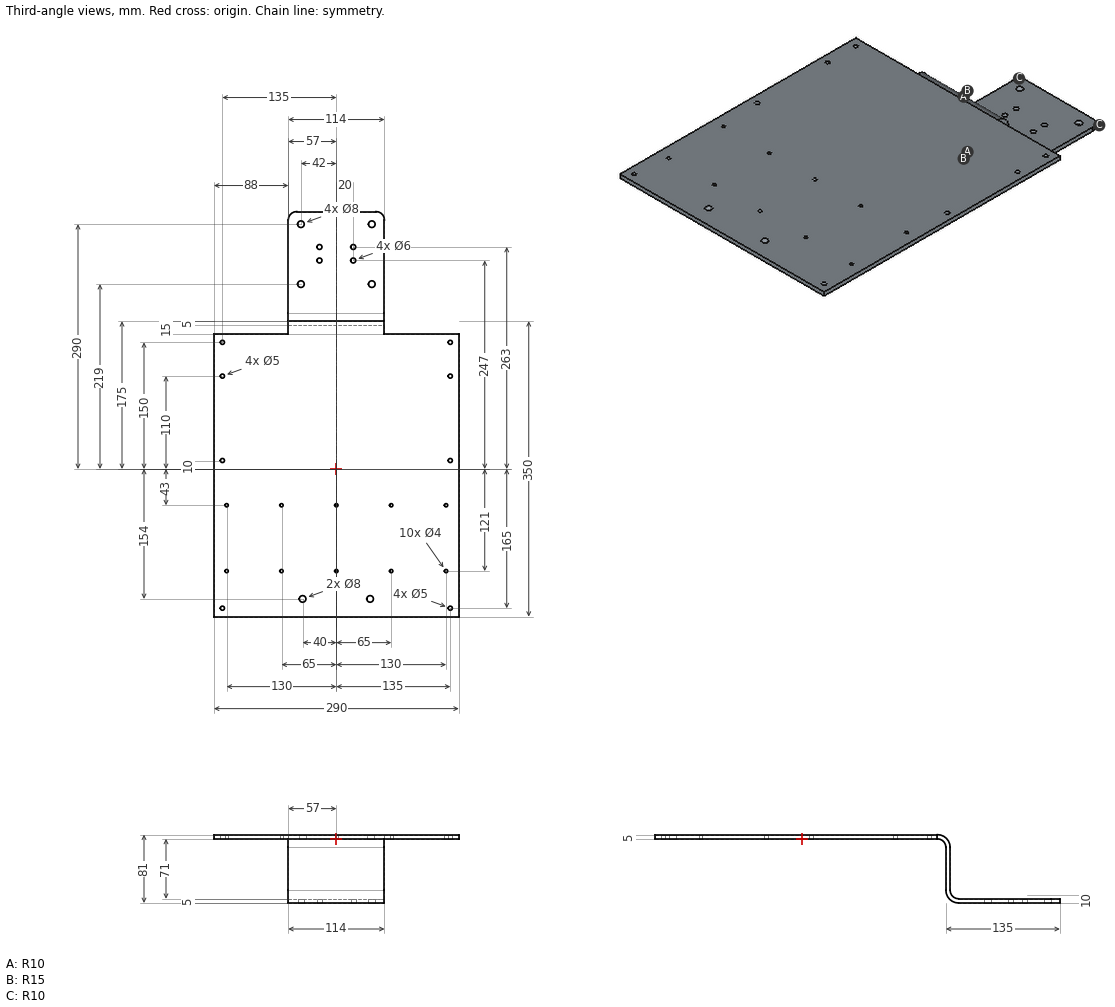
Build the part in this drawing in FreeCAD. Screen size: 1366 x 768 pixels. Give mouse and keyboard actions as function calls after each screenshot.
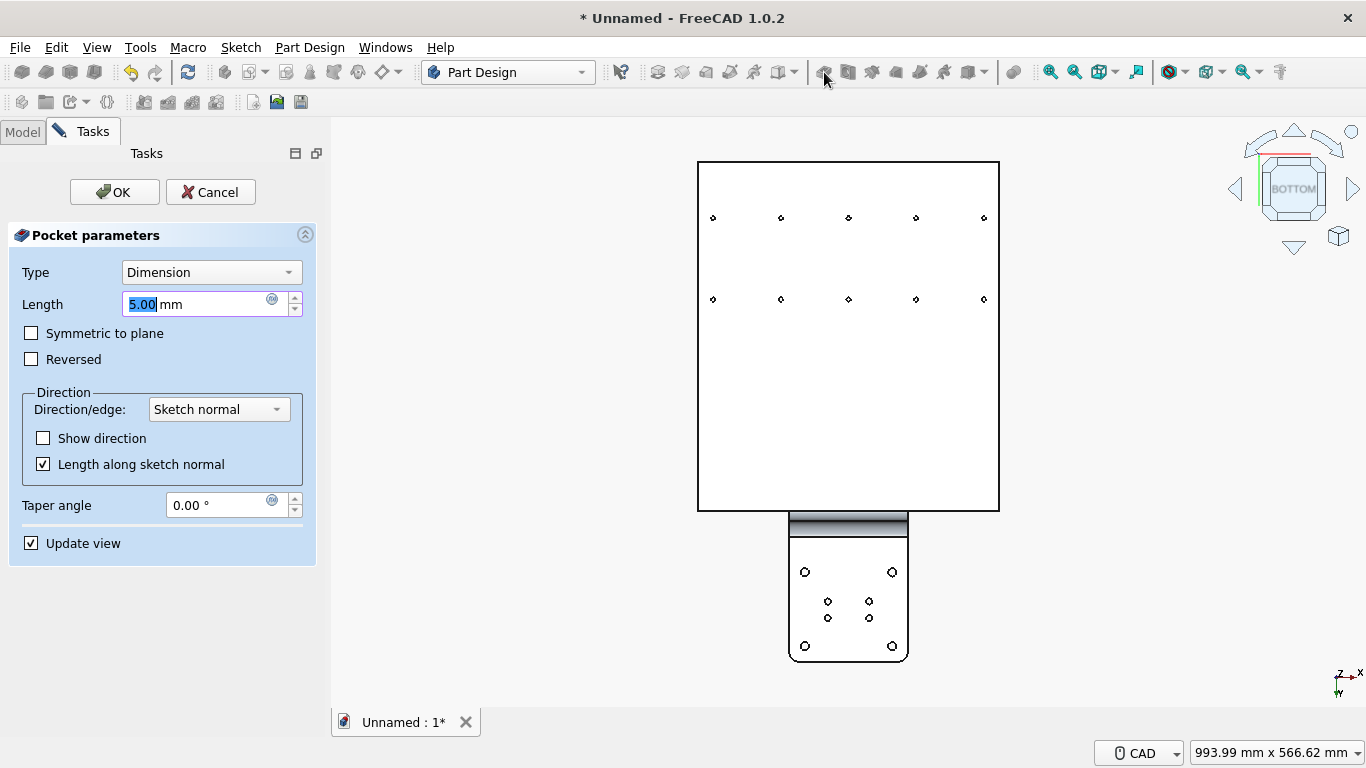
text(10)
key(Tab)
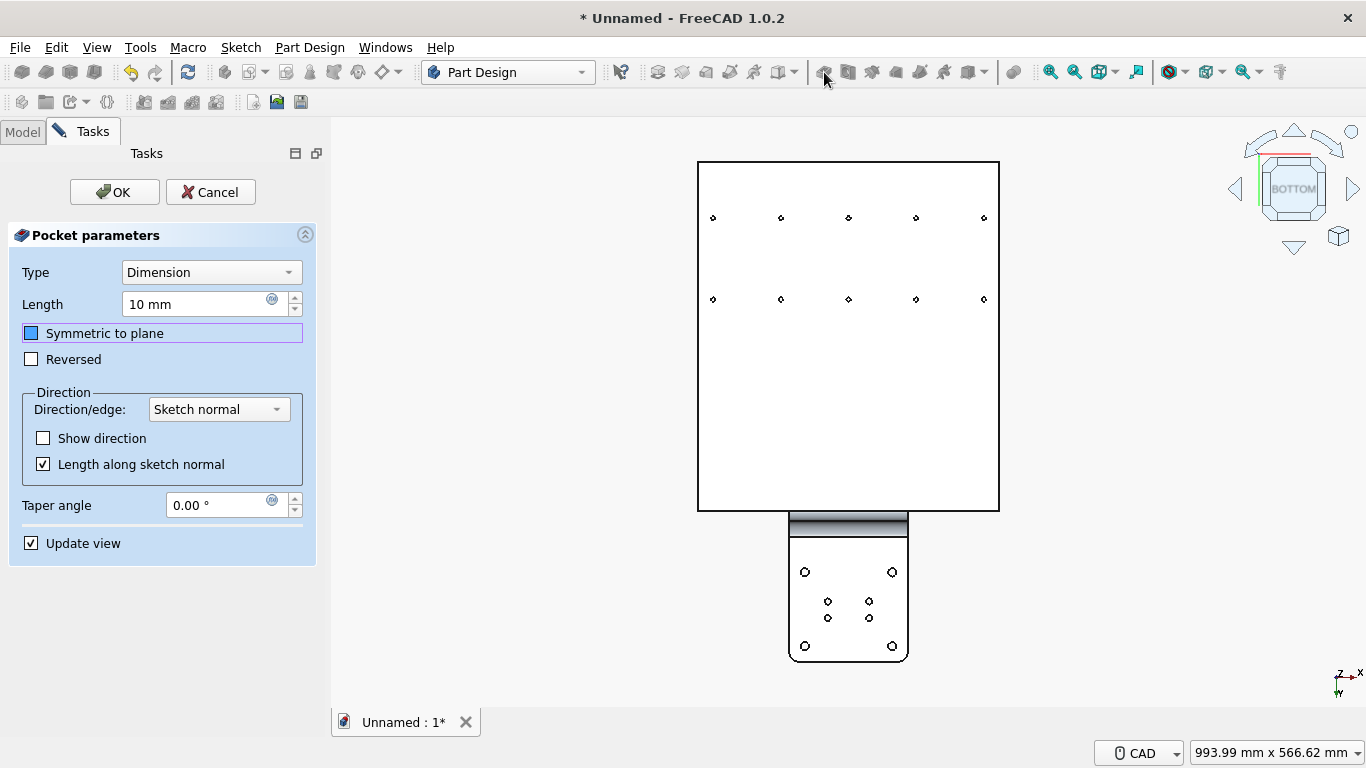
click(115, 192)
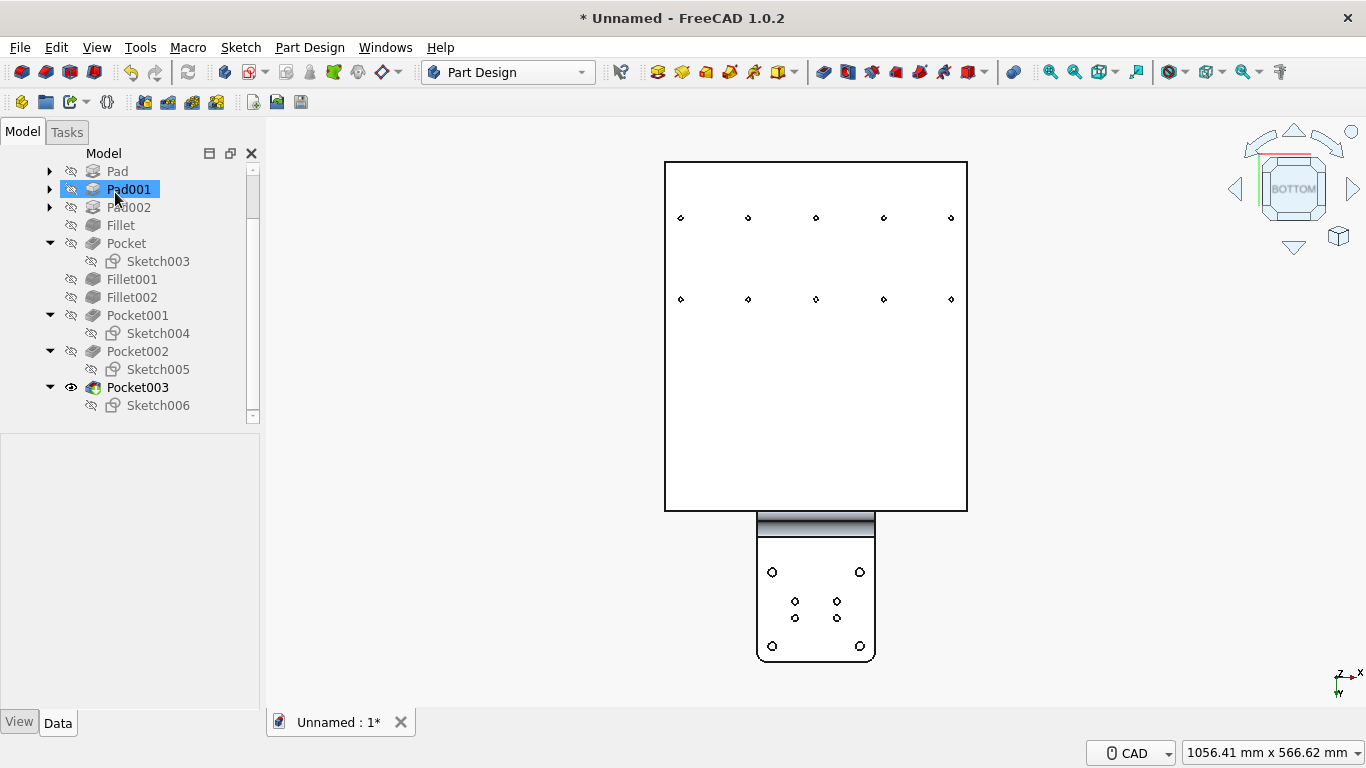
click(250, 72)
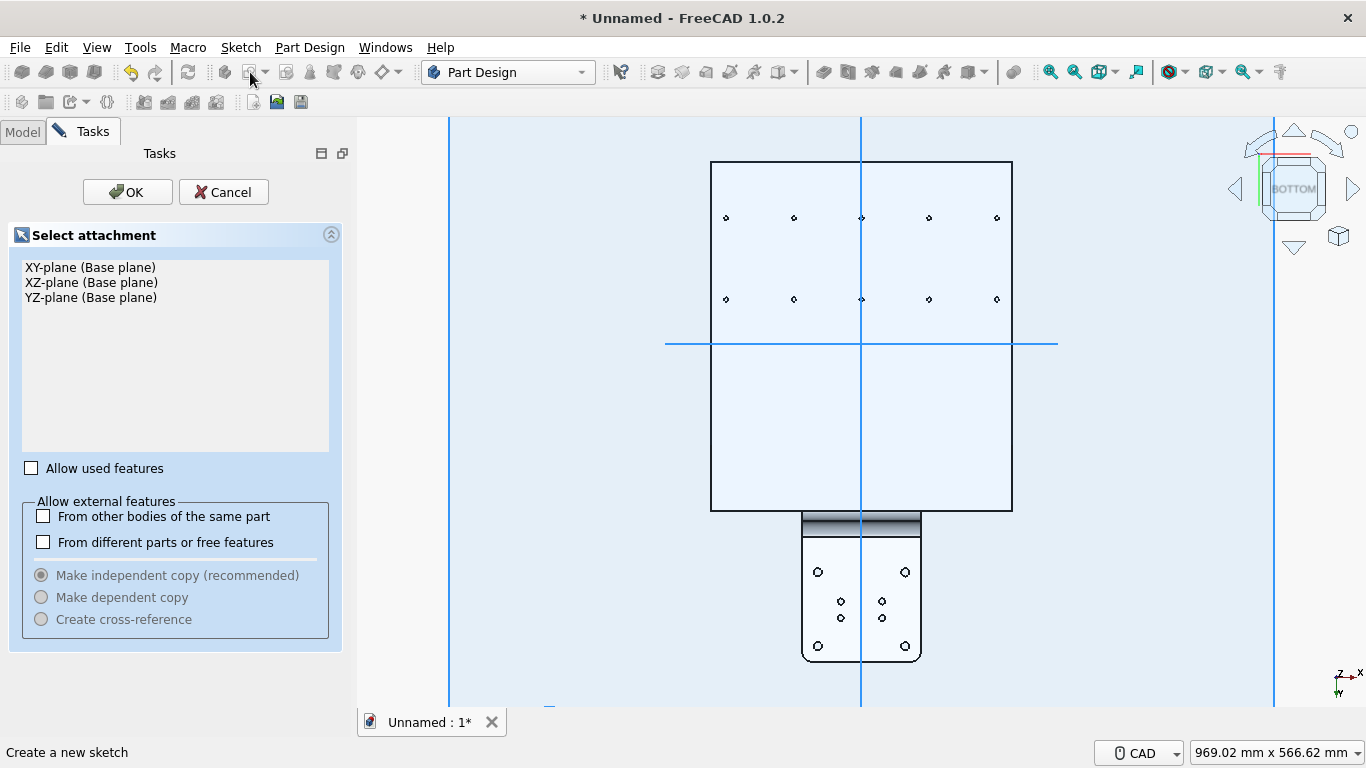
click(82, 268)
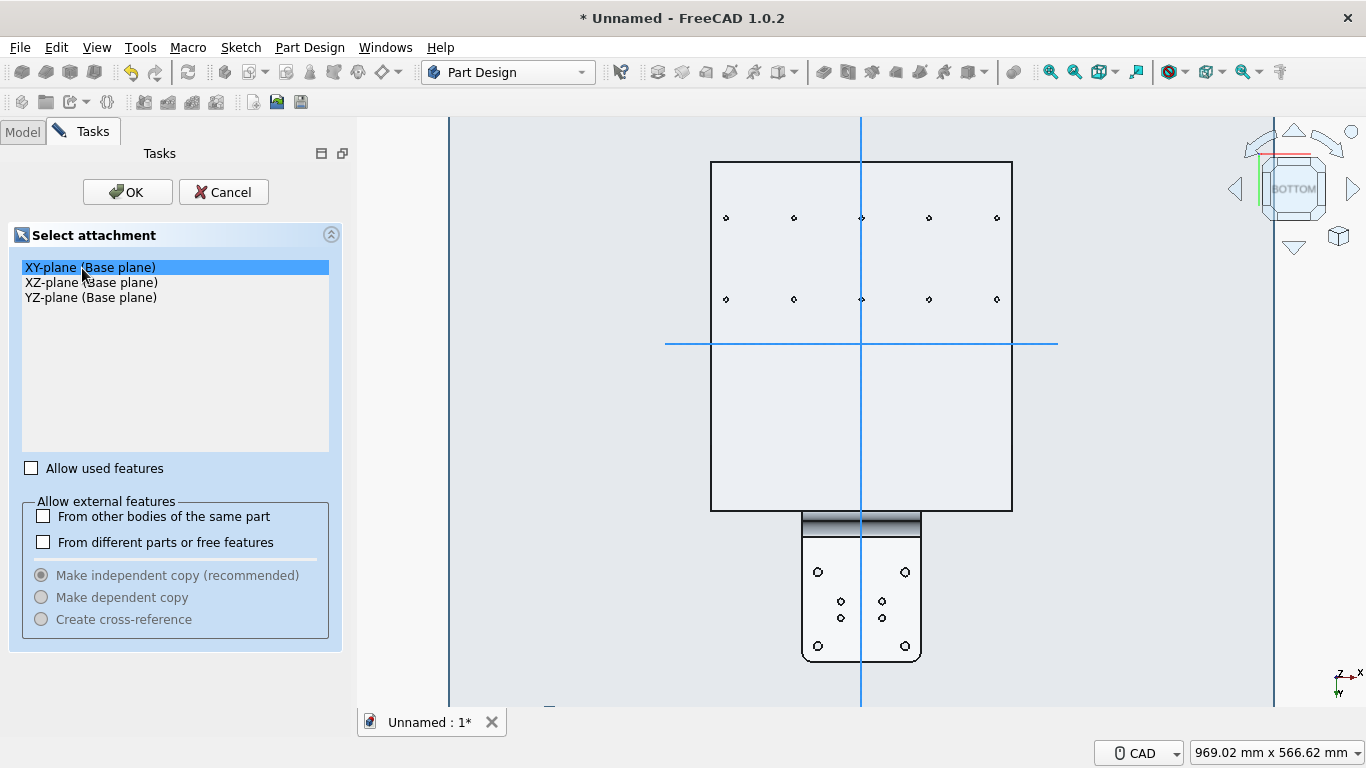
click(128, 192)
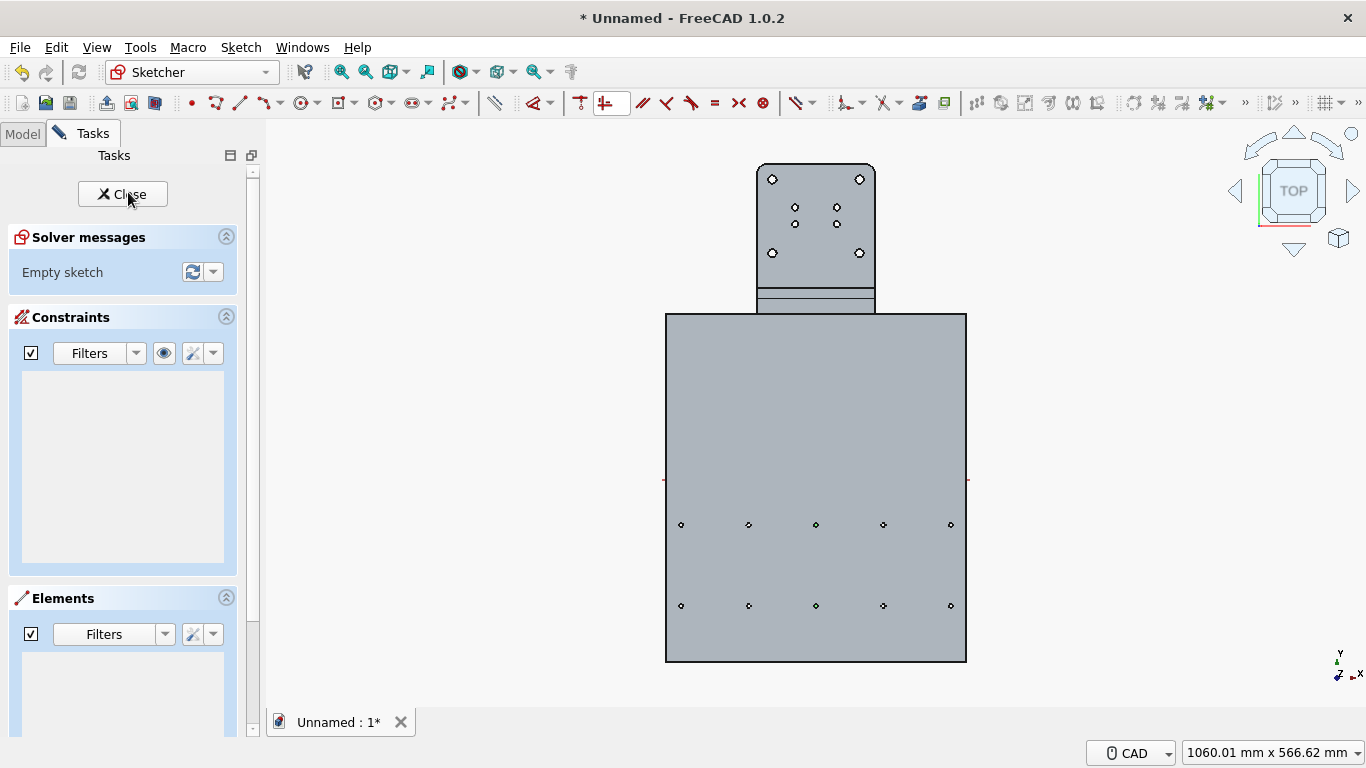
key(q)
key(s)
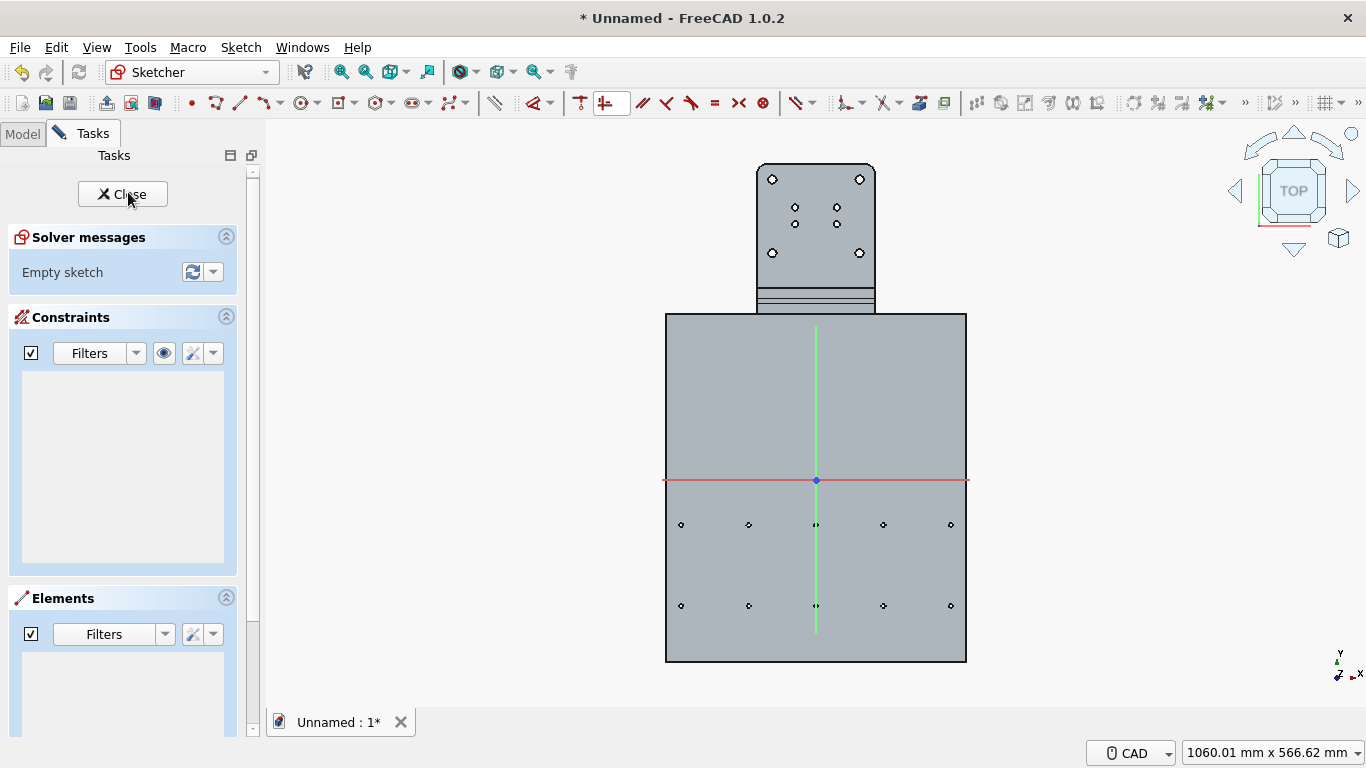
scroll(872, 679, up, 4)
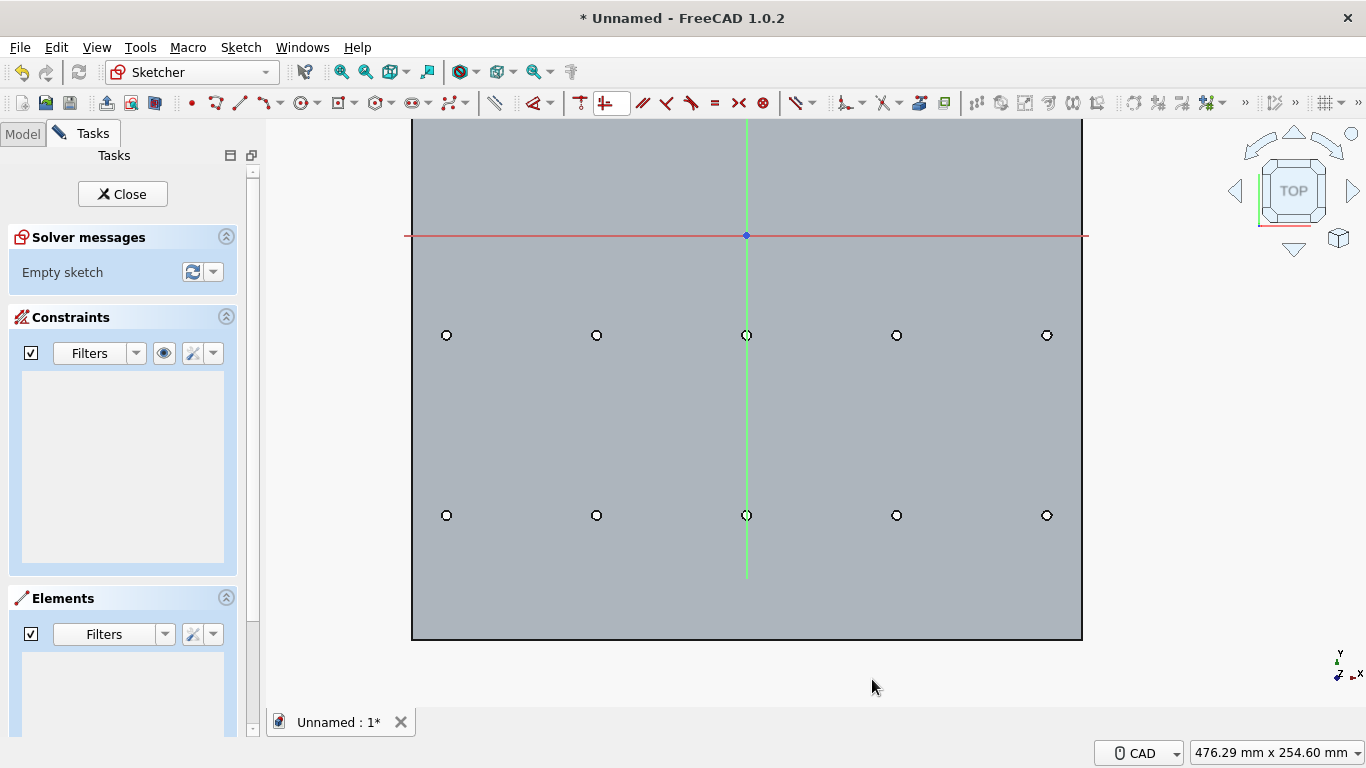
click(302, 104)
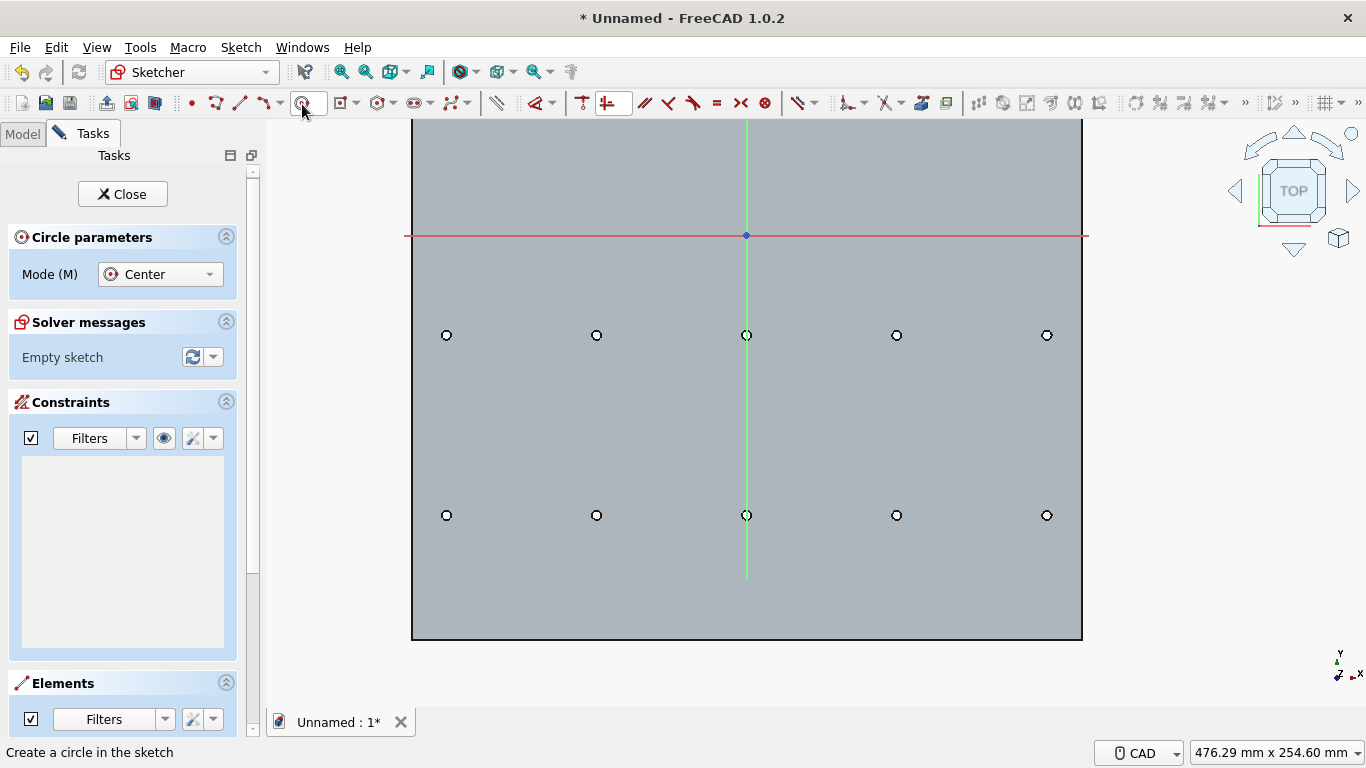
scroll(654, 592, up, 5)